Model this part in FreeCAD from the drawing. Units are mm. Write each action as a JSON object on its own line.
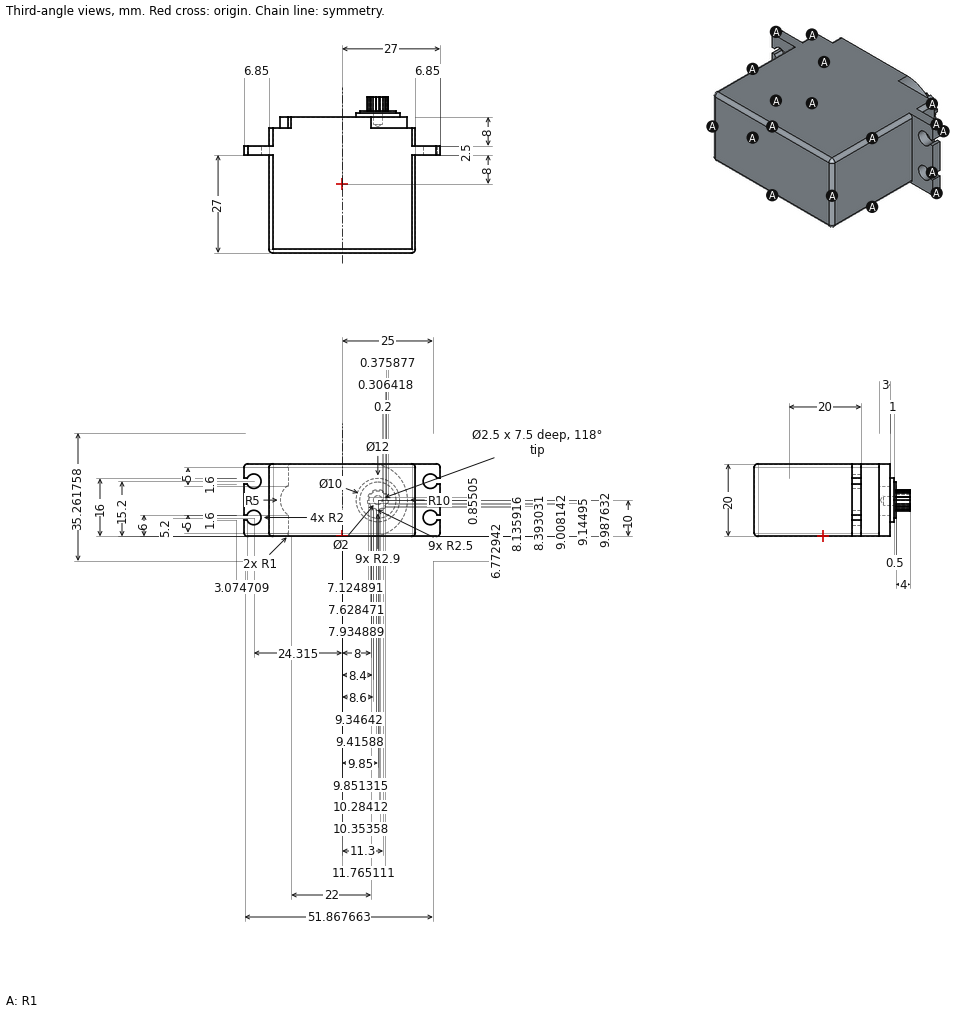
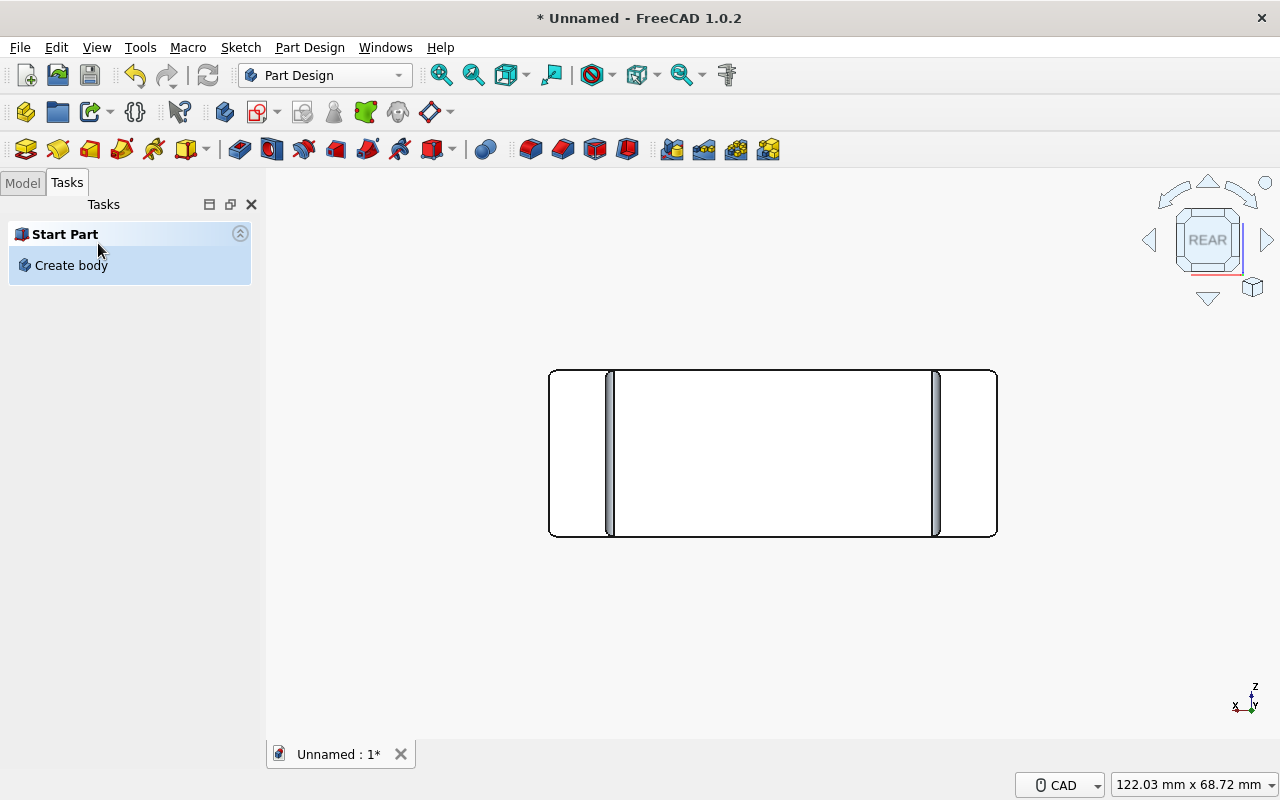
{"action": "left_click", "coordinate": [442, 76]}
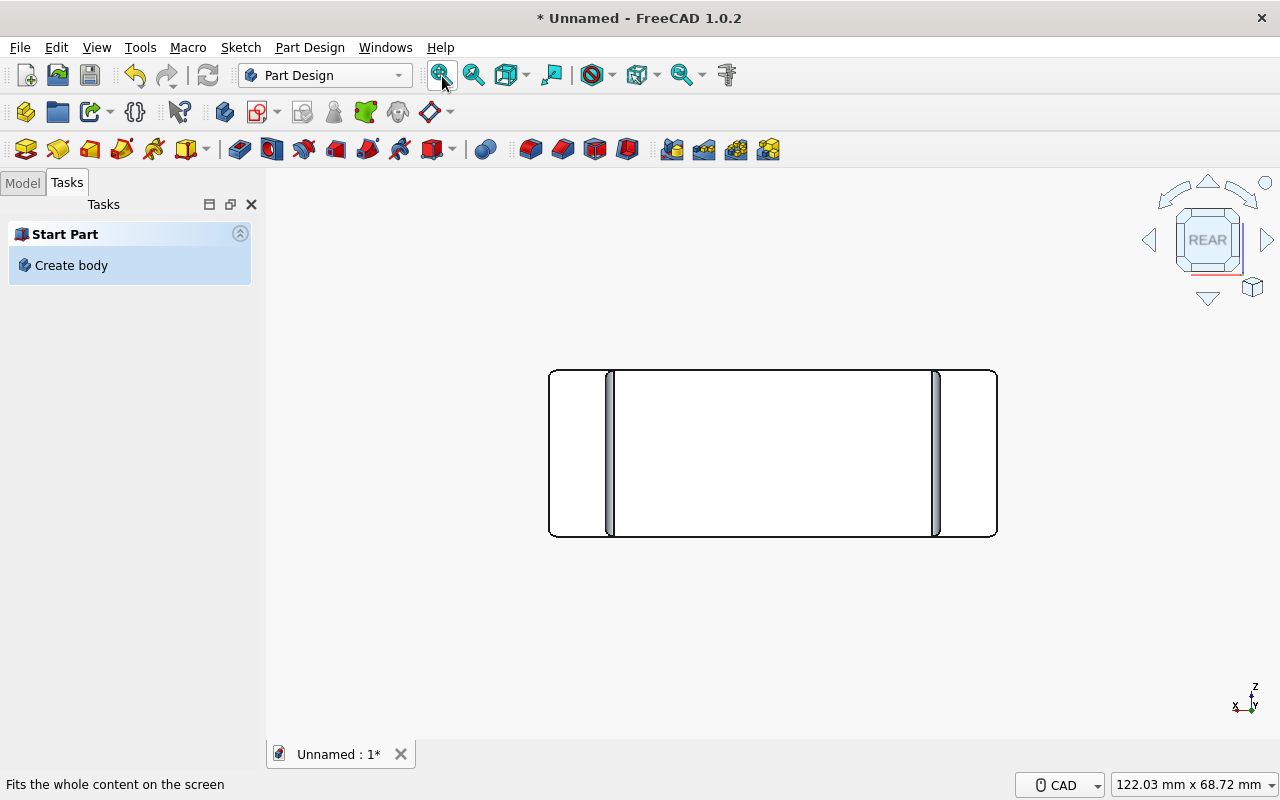
{"action": "left_click", "coordinate": [581, 405]}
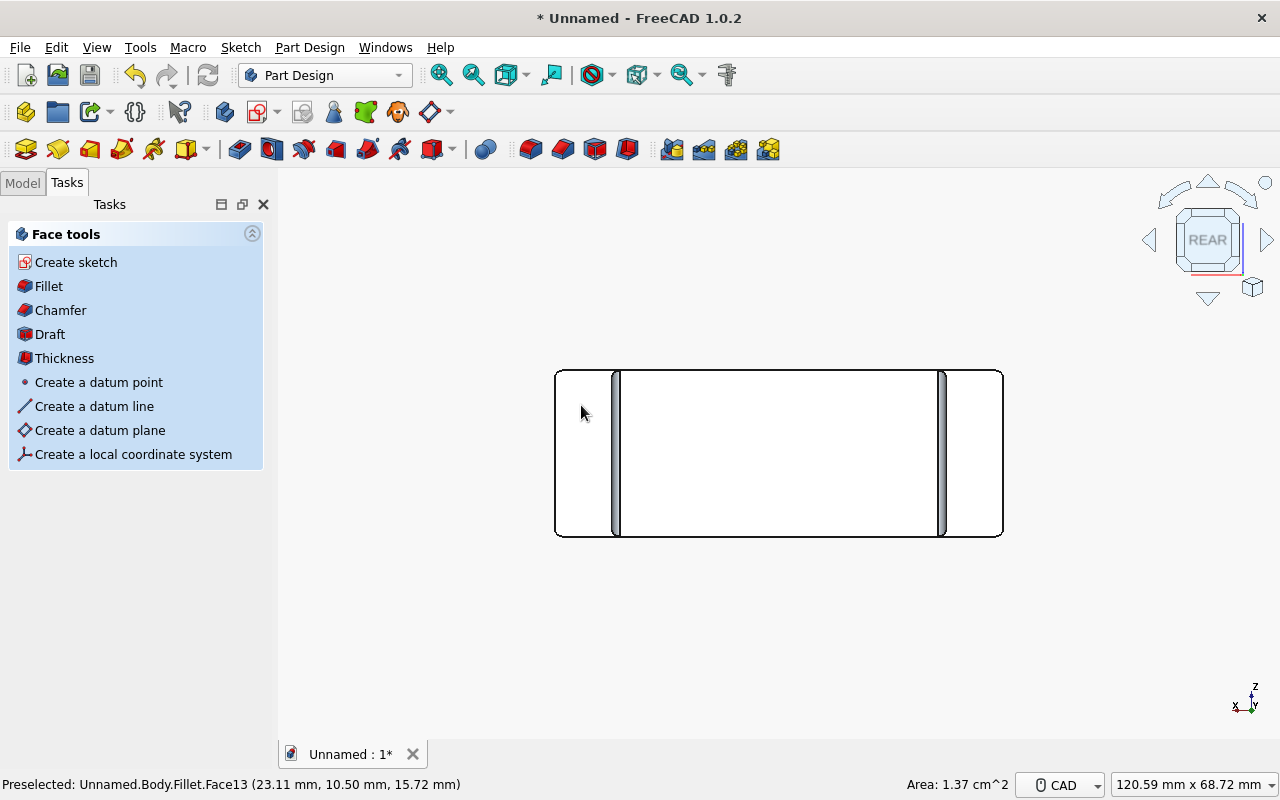
{"action": "left_click", "coordinate": [258, 112]}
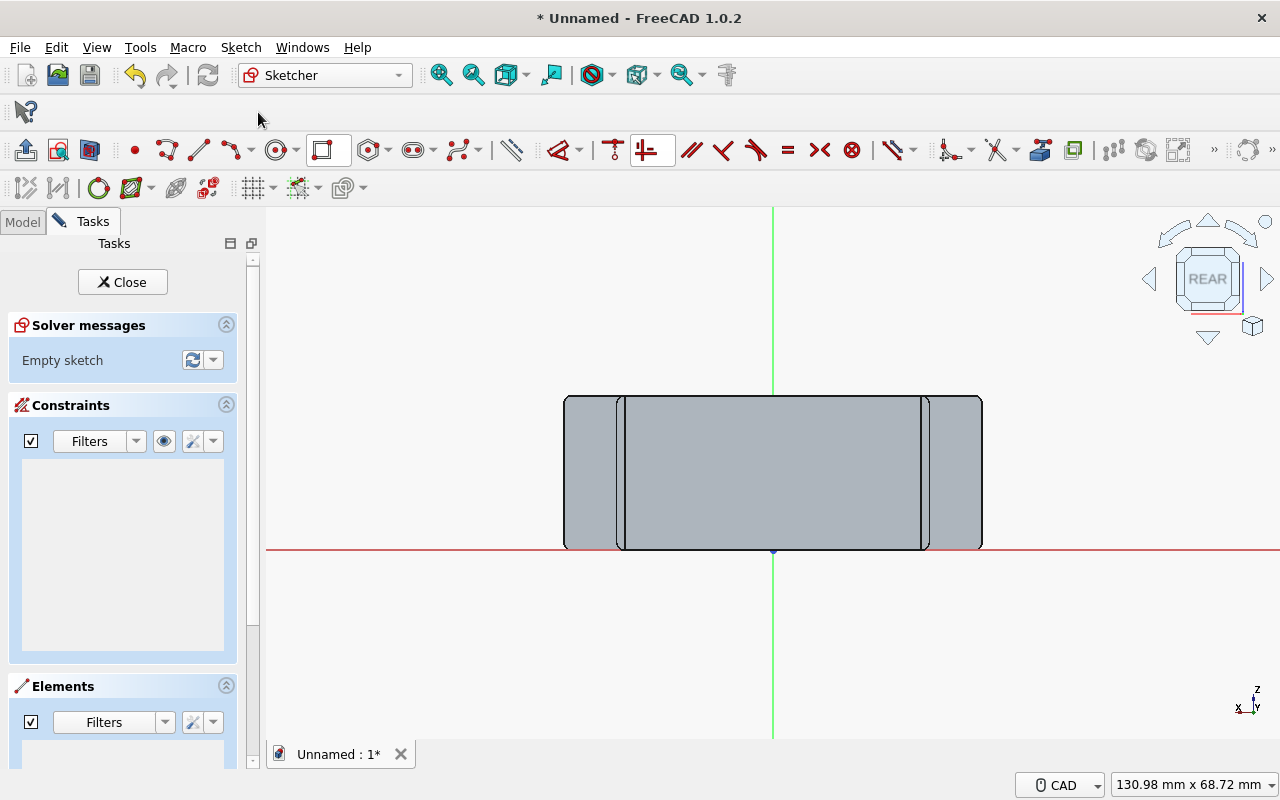
{"action": "key", "text": "g m"}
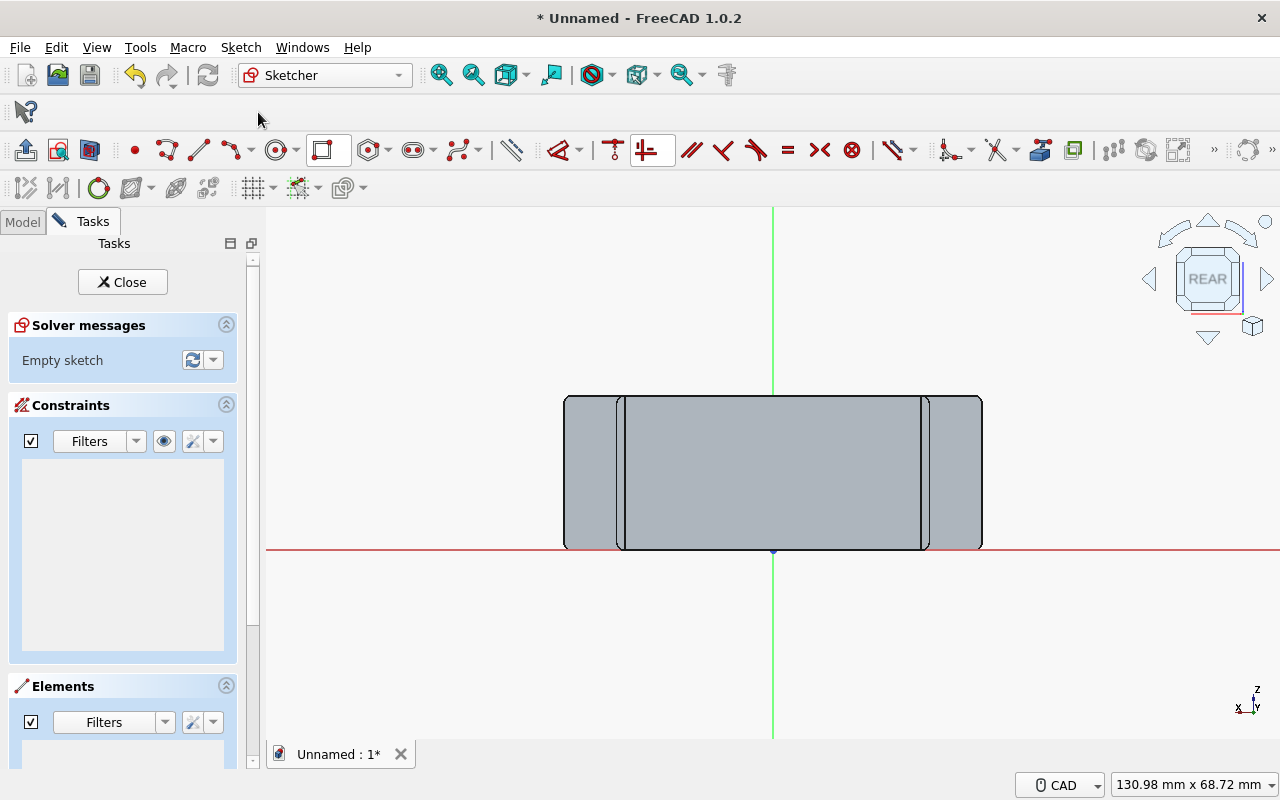
{"action": "left_click", "coordinate": [975, 516]}
{"action": "left_click", "coordinate": [999, 516]}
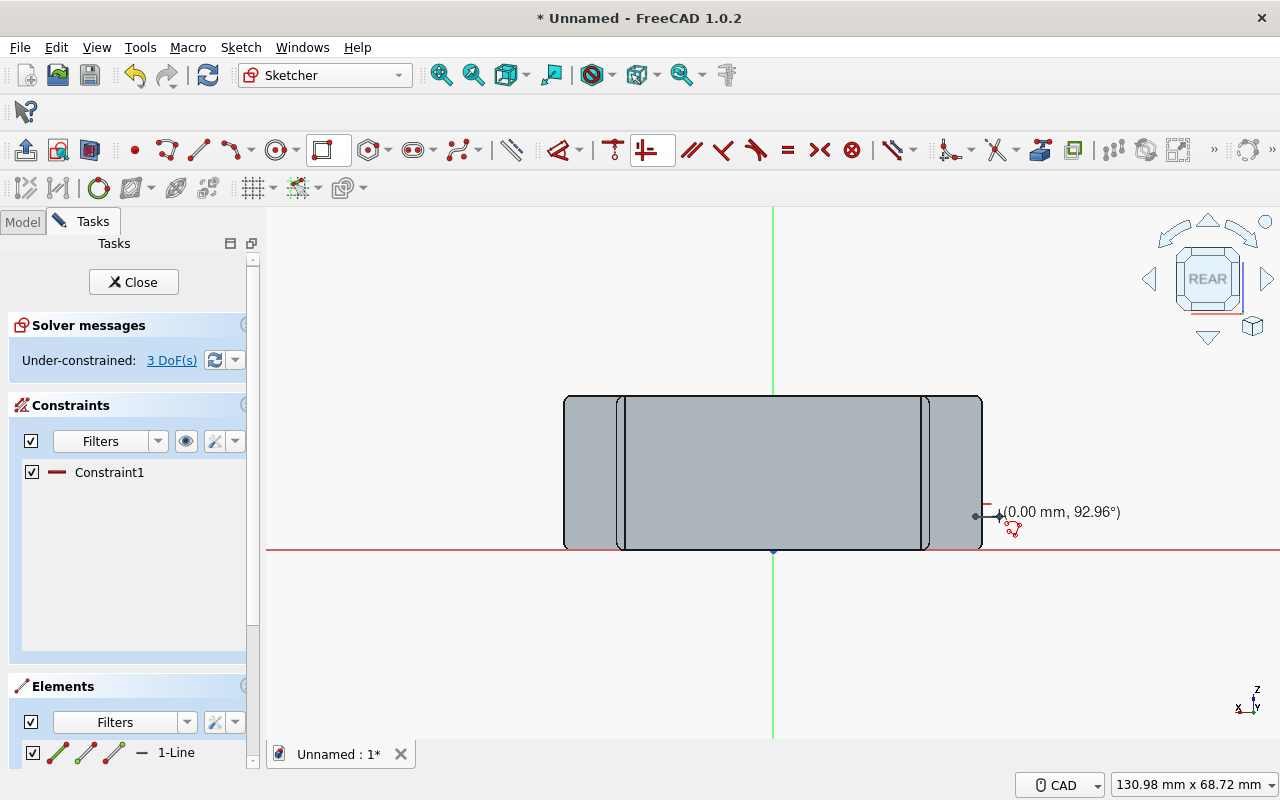
{"action": "scroll", "coordinate": [999, 504], "scroll_direction": "up", "scroll_amount": 2}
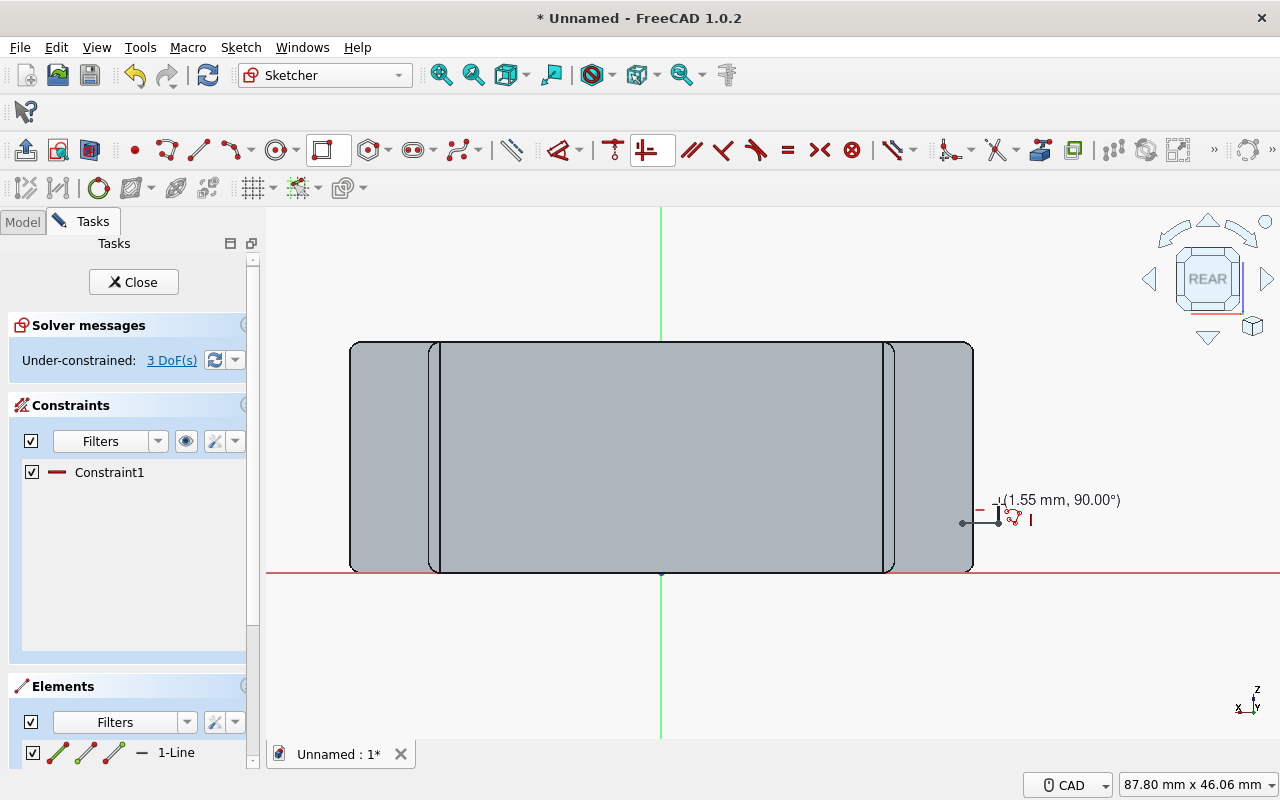
{"action": "left_click", "coordinate": [999, 504]}
{"action": "left_click", "coordinate": [963, 504]}
{"action": "right_click", "coordinate": [963, 504]}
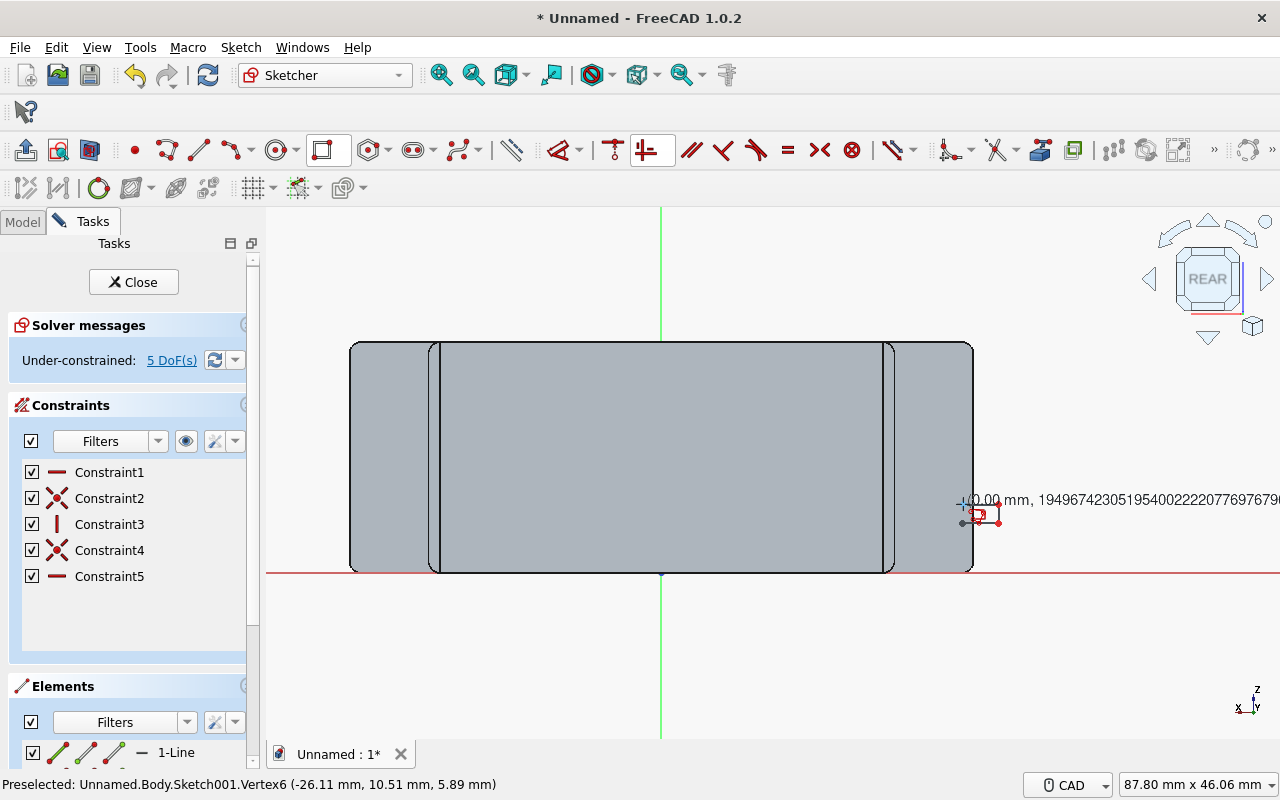
{"action": "key", "text": "g 3 a"}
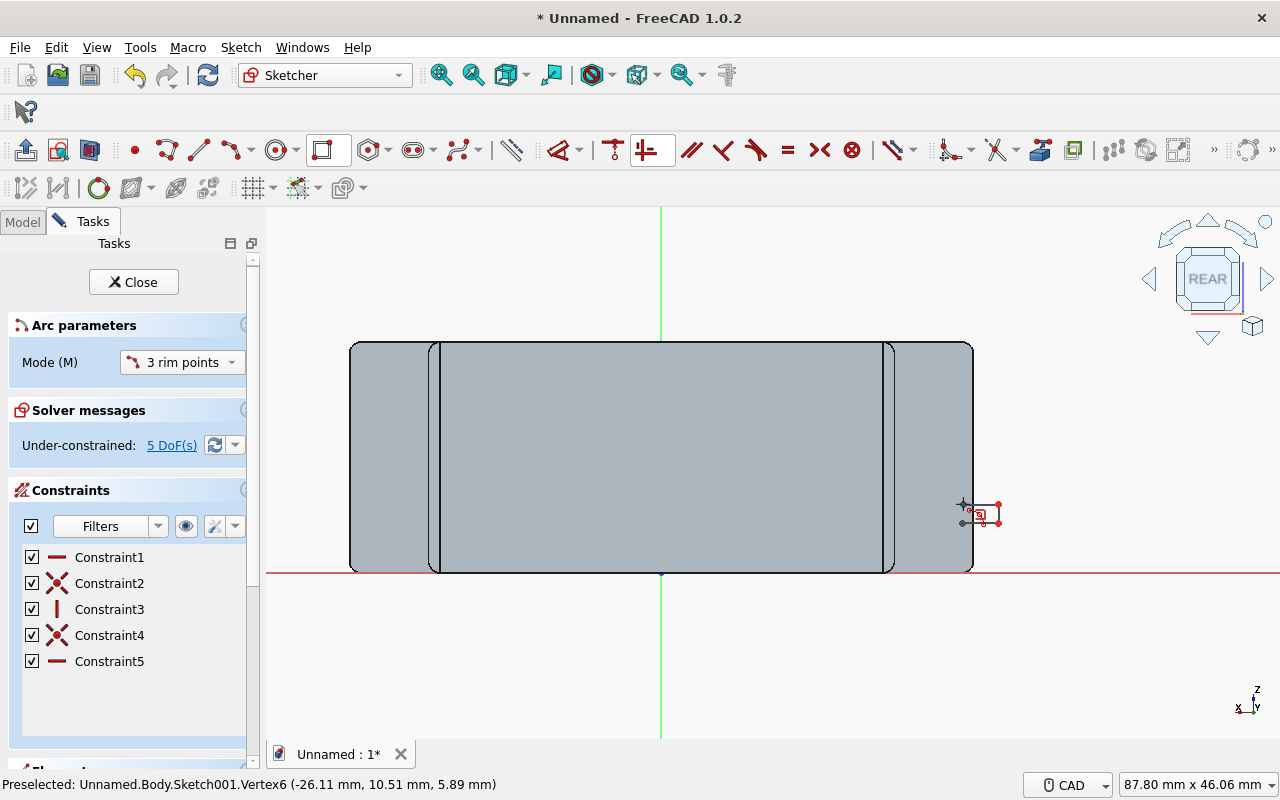
{"action": "left_click", "coordinate": [963, 505]}
{"action": "left_click", "coordinate": [963, 523]}
{"action": "left_click", "coordinate": [919, 513]}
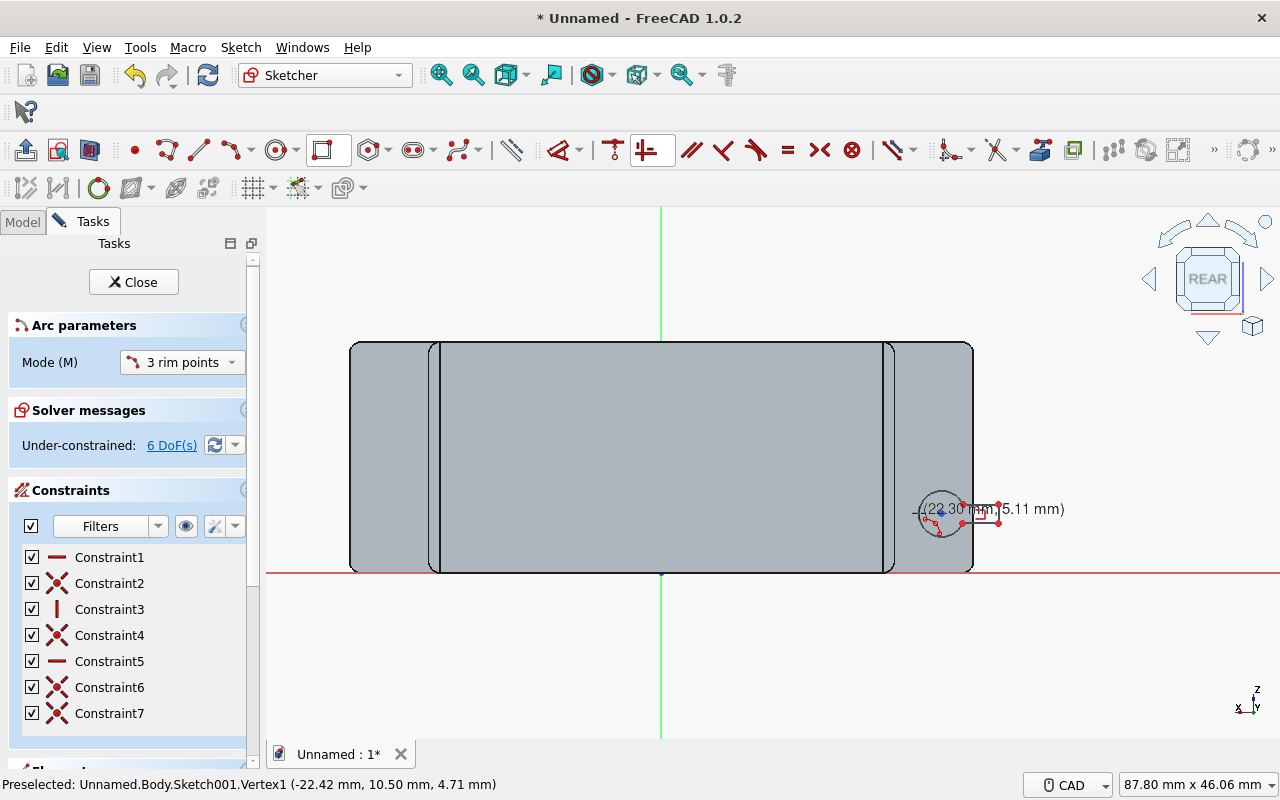
{"action": "left_click", "coordinate": [168, 150]}